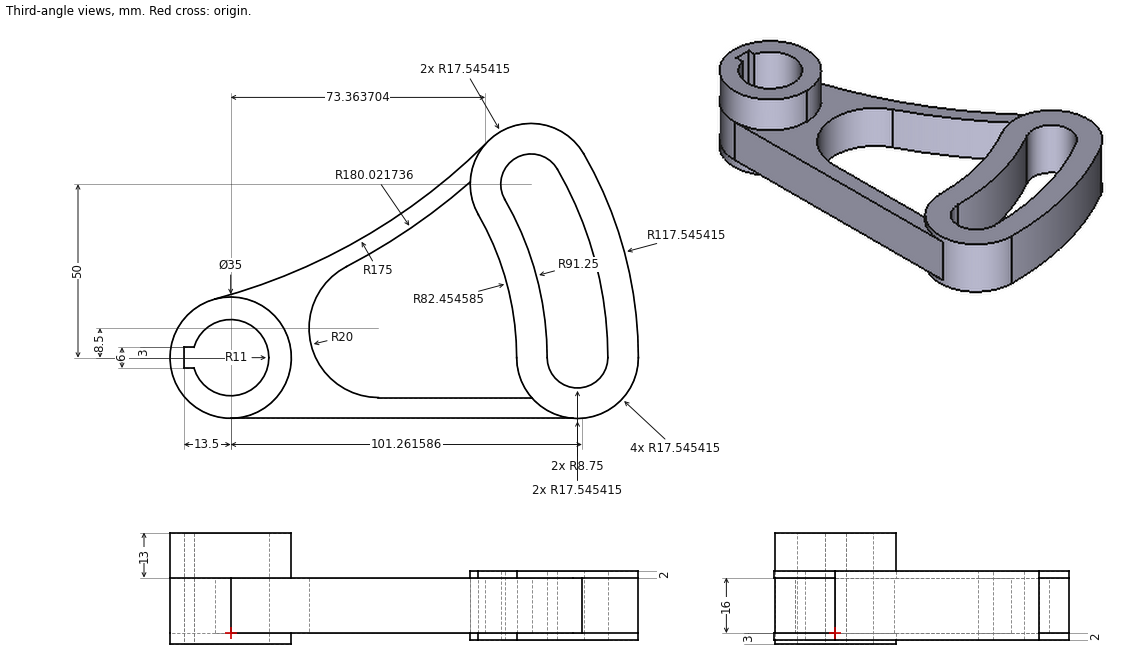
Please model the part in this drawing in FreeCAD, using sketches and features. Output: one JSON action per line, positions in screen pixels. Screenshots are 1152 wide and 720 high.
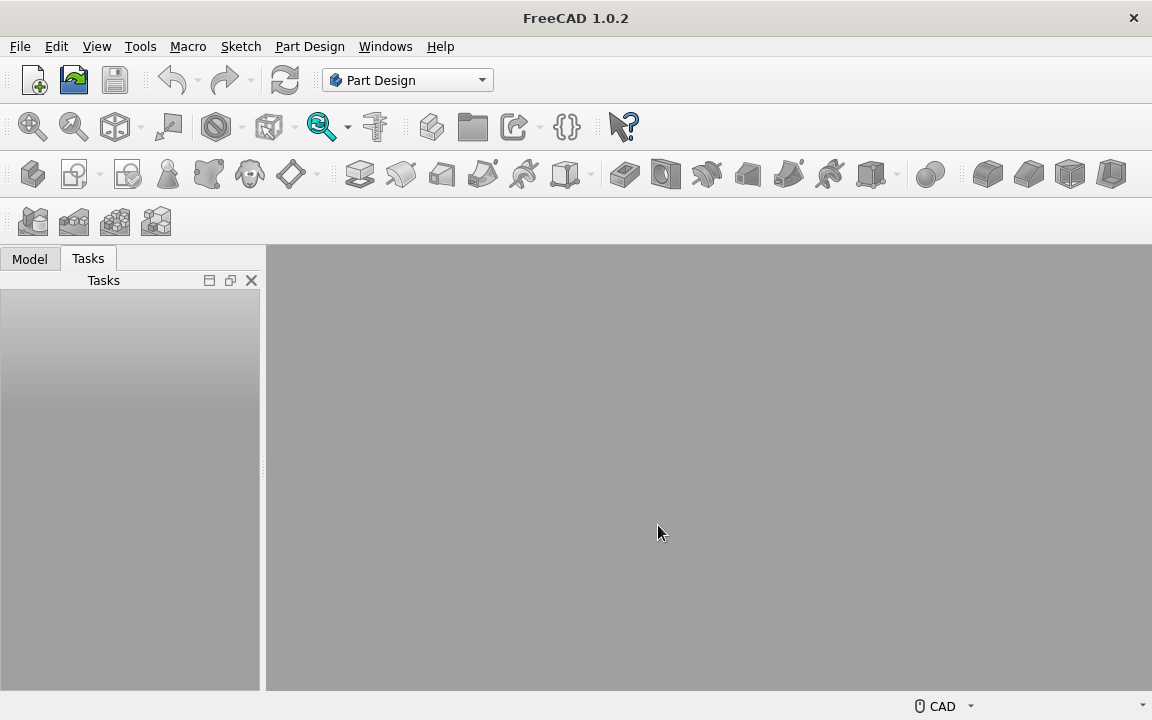
{"action": "left_click", "coordinate": [33, 80]}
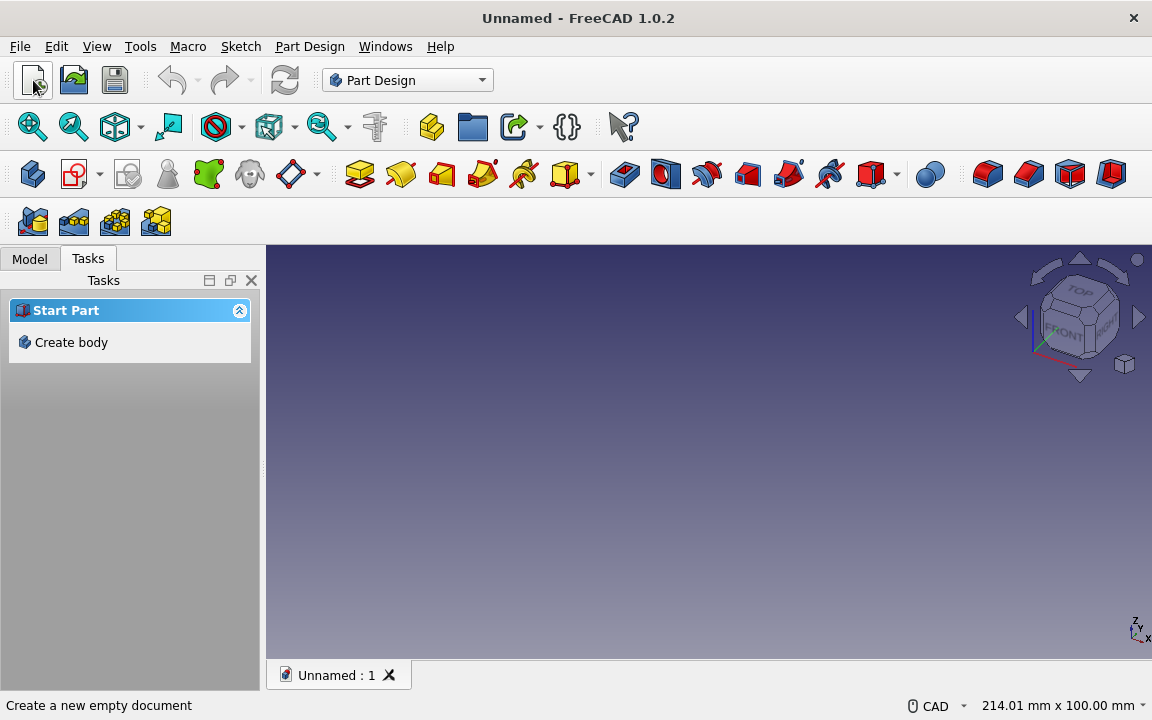
{"action": "left_click", "coordinate": [74, 174]}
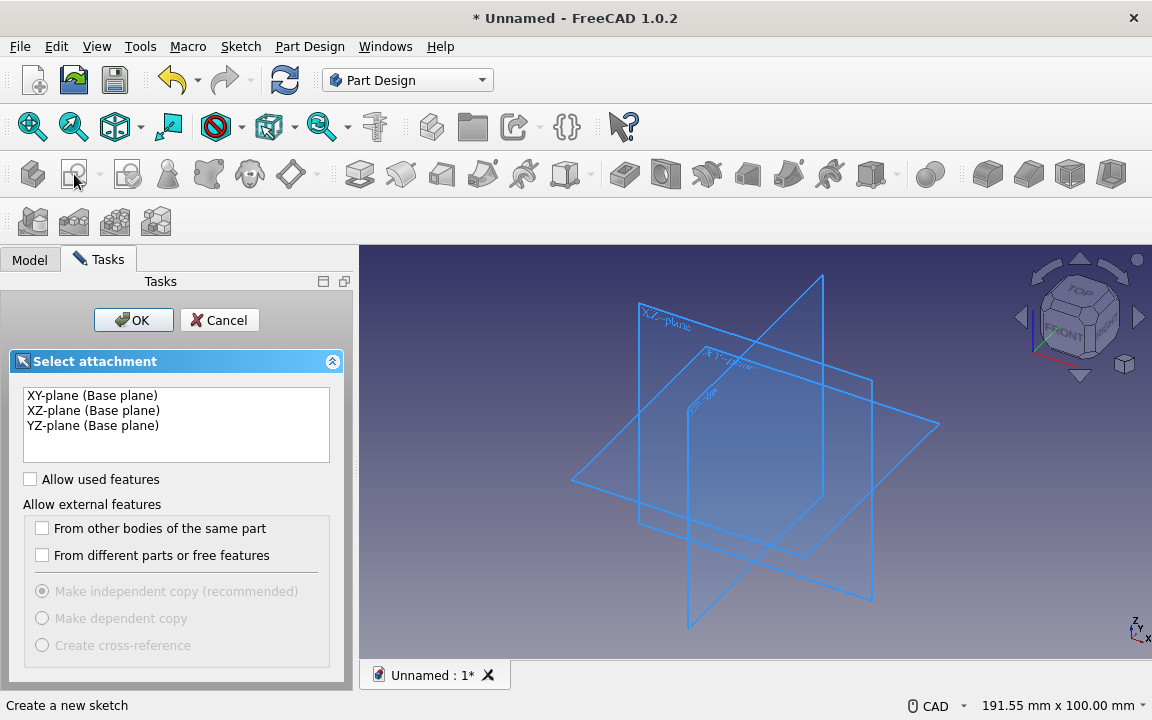
{"action": "left_click", "coordinate": [84, 396]}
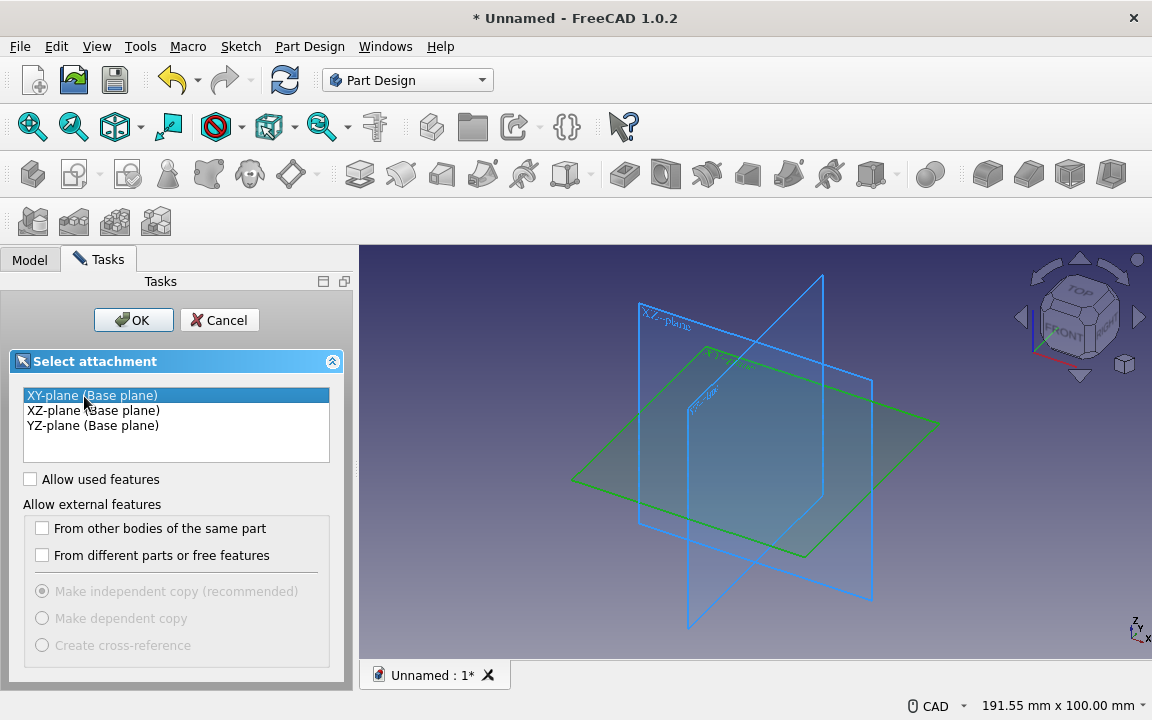
{"action": "left_click", "coordinate": [134, 320]}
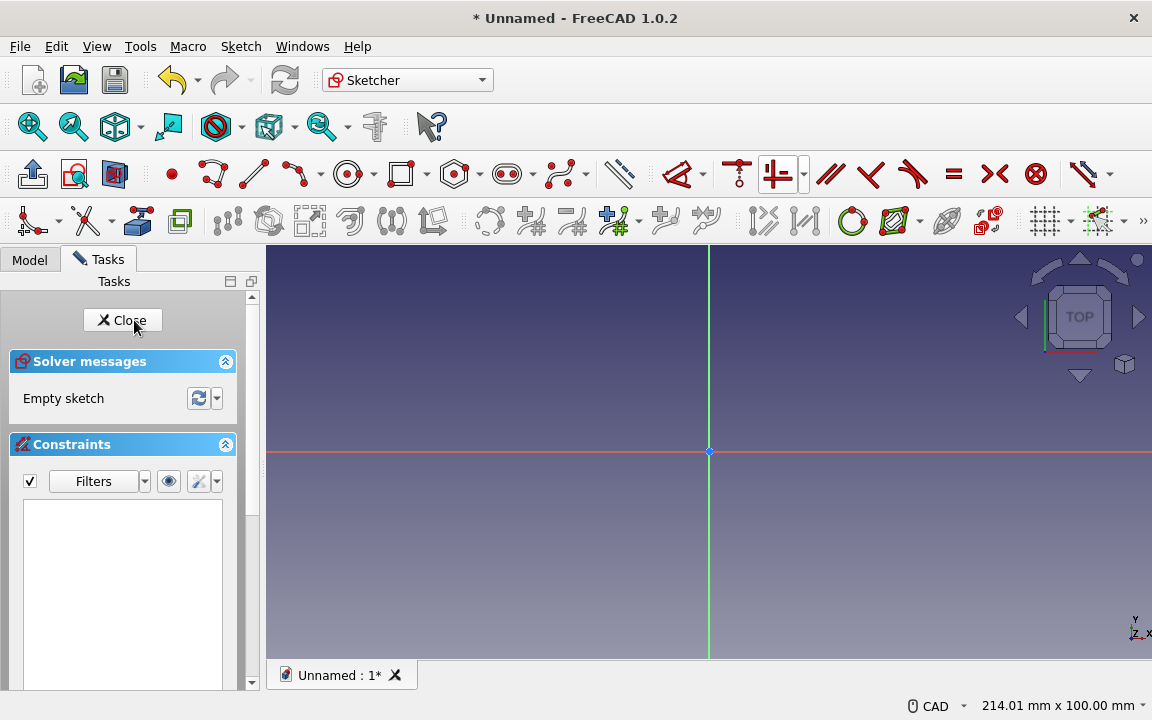
{"action": "scroll", "coordinate": [294, 631], "scroll_direction": "down", "scroll_amount": 2}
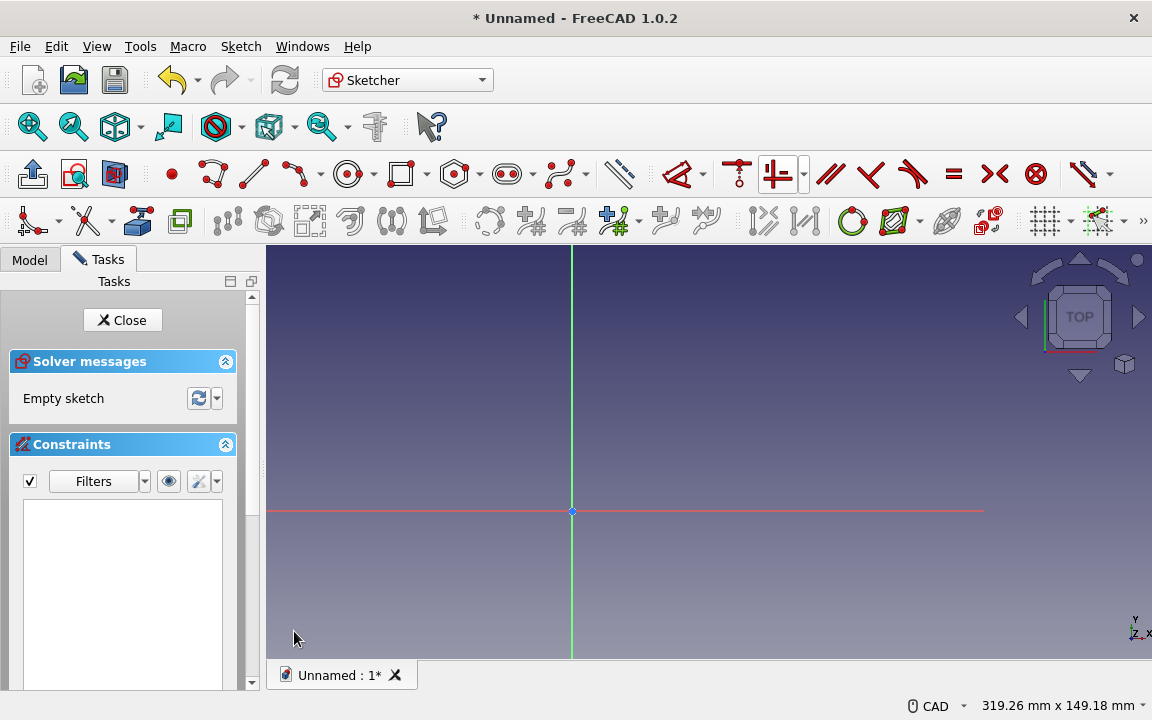
{"action": "left_click", "coordinate": [254, 174]}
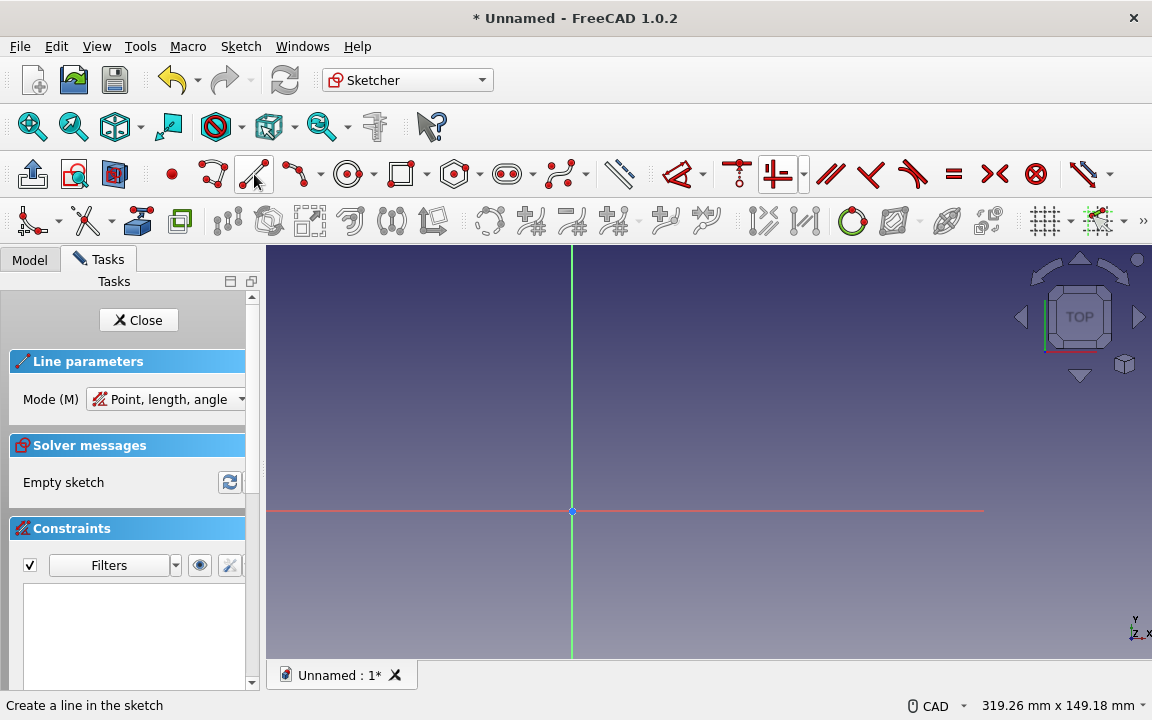
{"action": "left_click", "coordinate": [572, 560]}
{"action": "left_click", "coordinate": [853, 560]}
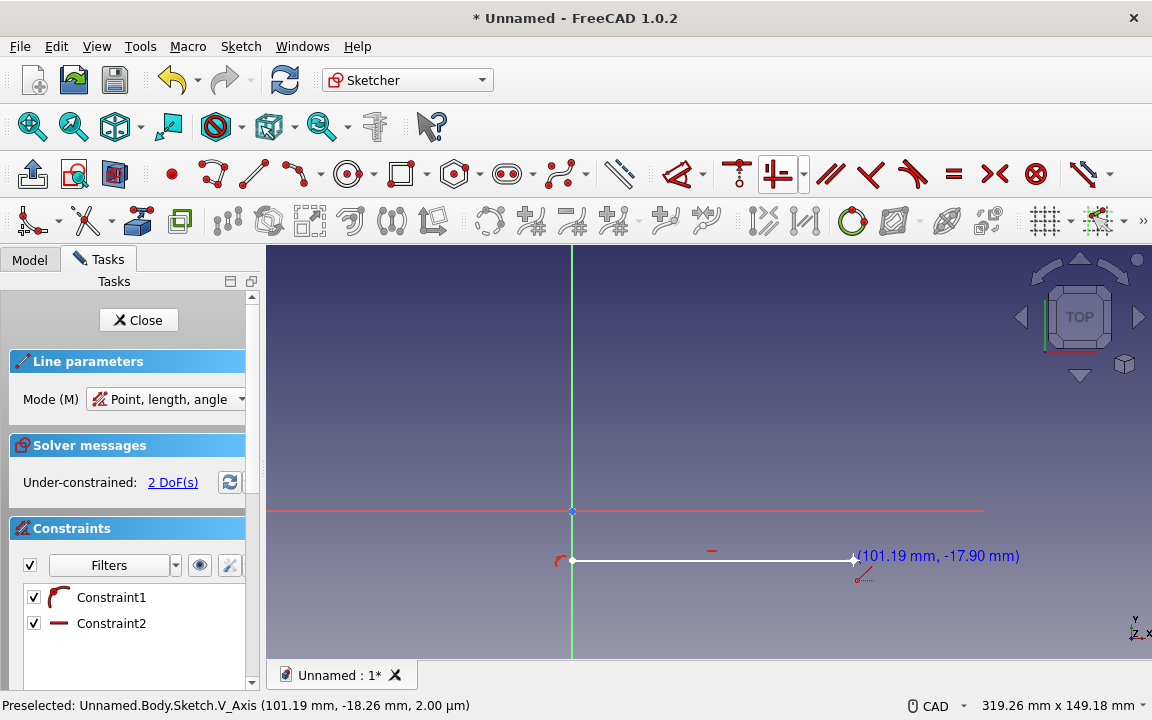
{"action": "left_click", "coordinate": [294, 174]}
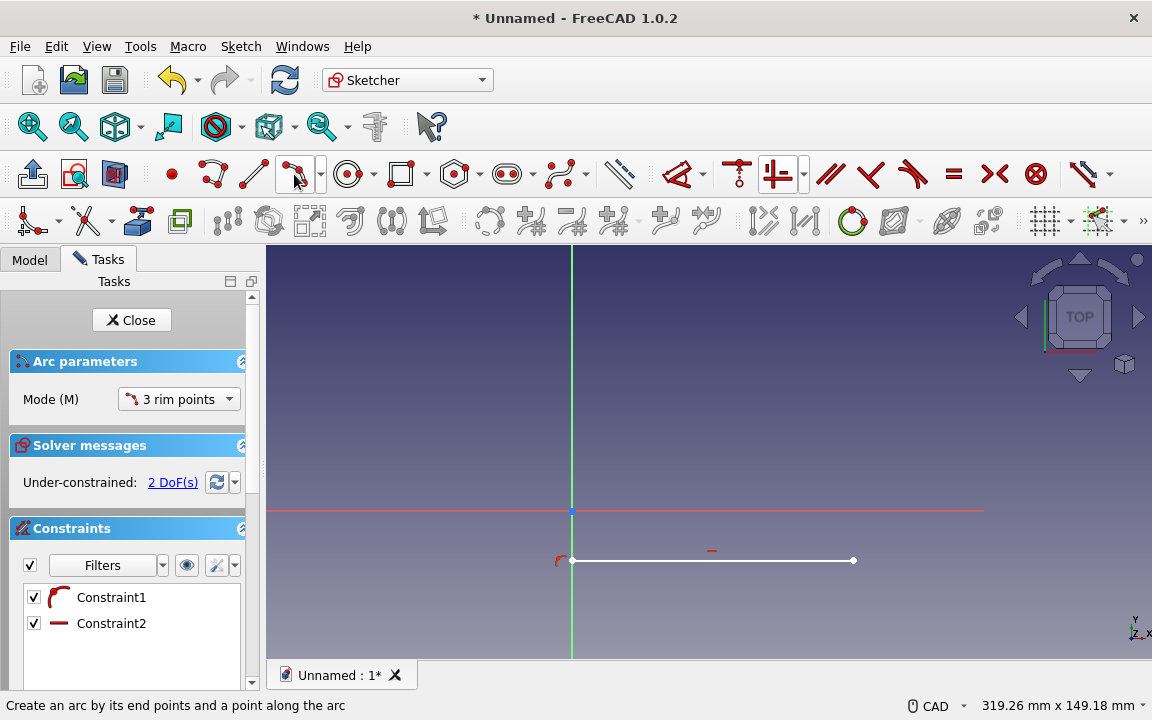
{"action": "left_click", "coordinate": [853, 561]}
{"action": "left_click", "coordinate": [898, 511]}
{"action": "left_click", "coordinate": [885, 544]}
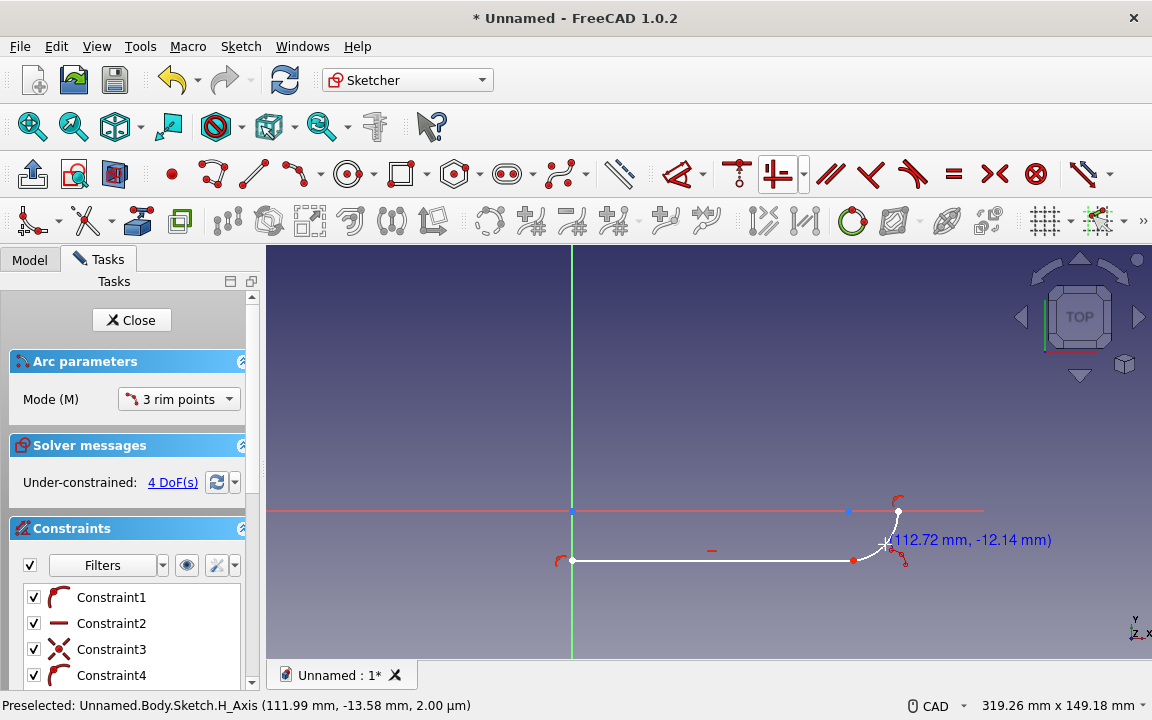
{"action": "left_click", "coordinate": [898, 511]}
{"action": "left_click", "coordinate": [855, 348]}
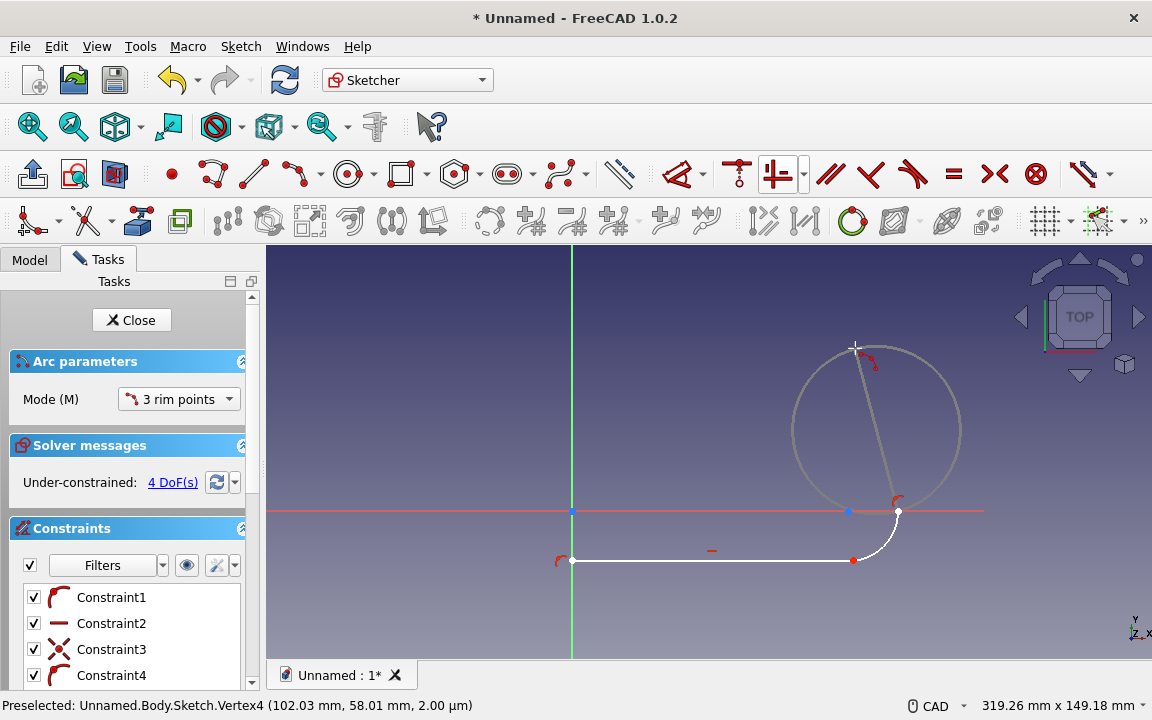
{"action": "scroll", "coordinate": [887, 427], "scroll_direction": "up", "scroll_amount": 2}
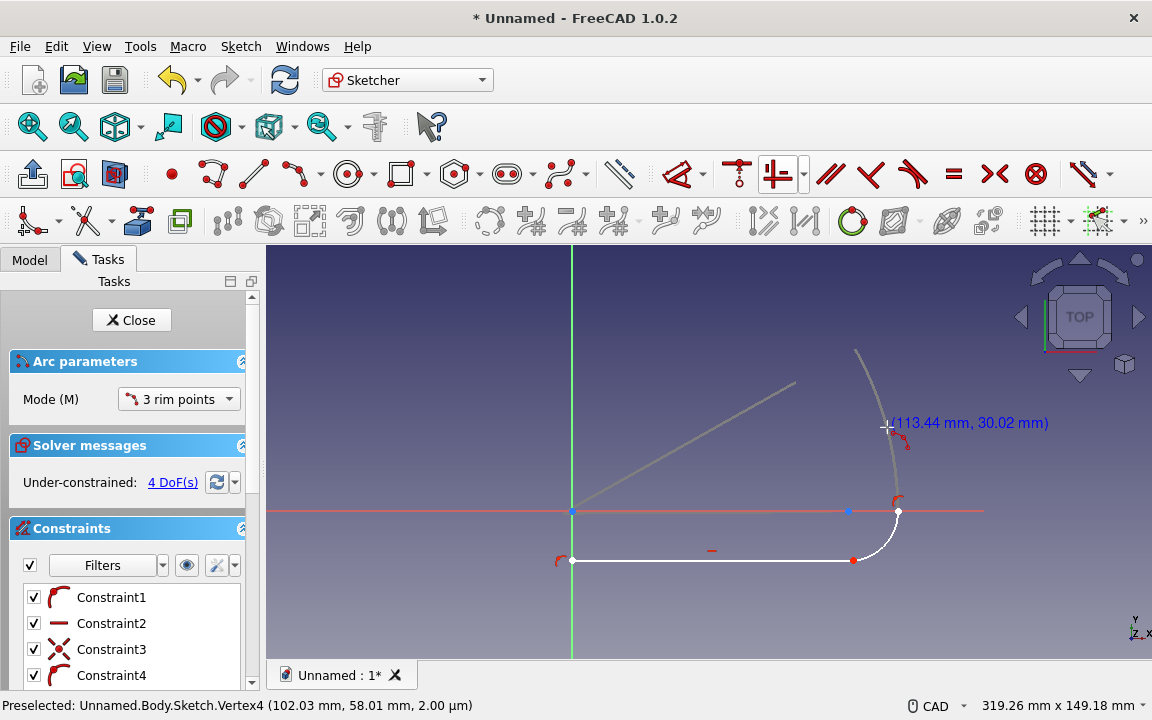
{"action": "left_click", "coordinate": [887, 427]}